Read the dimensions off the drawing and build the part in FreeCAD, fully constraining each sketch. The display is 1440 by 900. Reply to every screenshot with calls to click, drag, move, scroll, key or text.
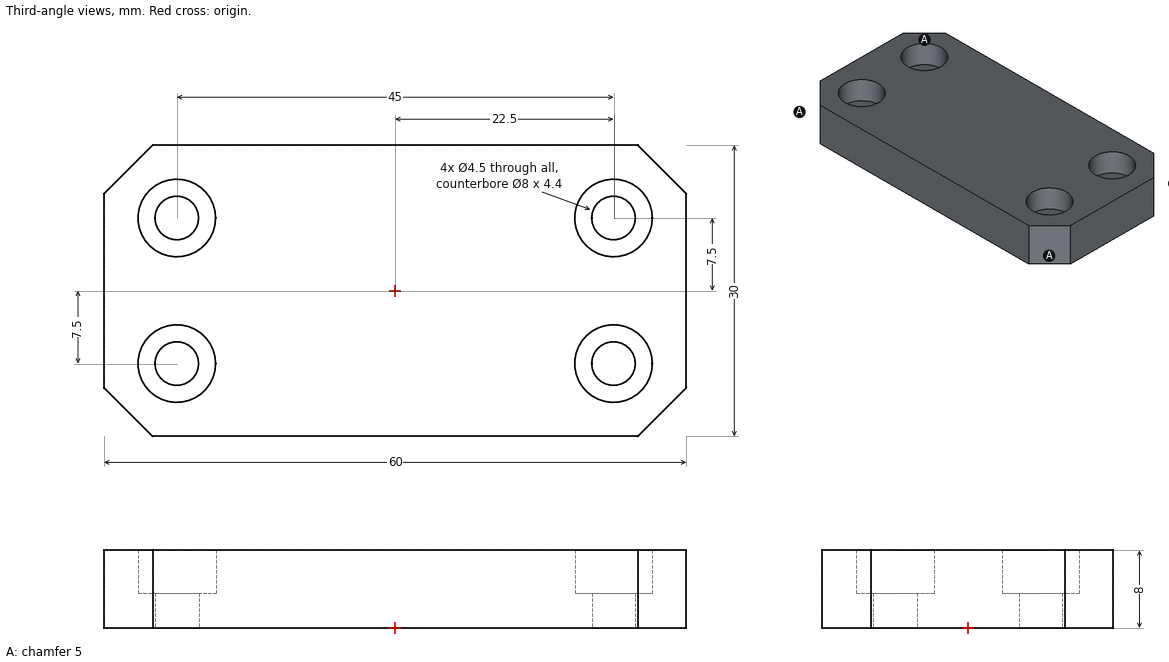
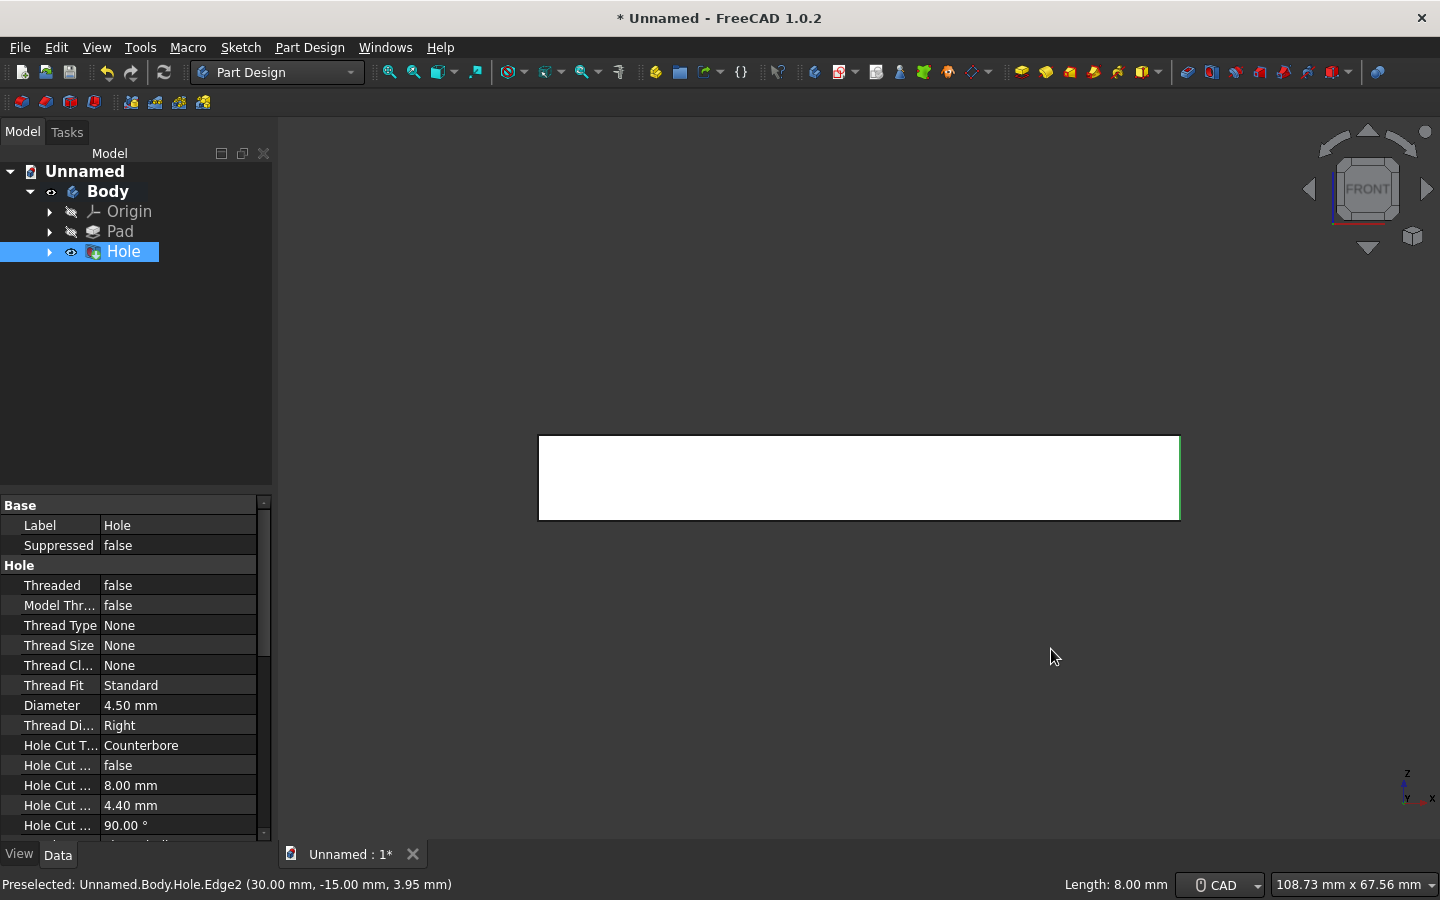
click(538, 477, ctrl)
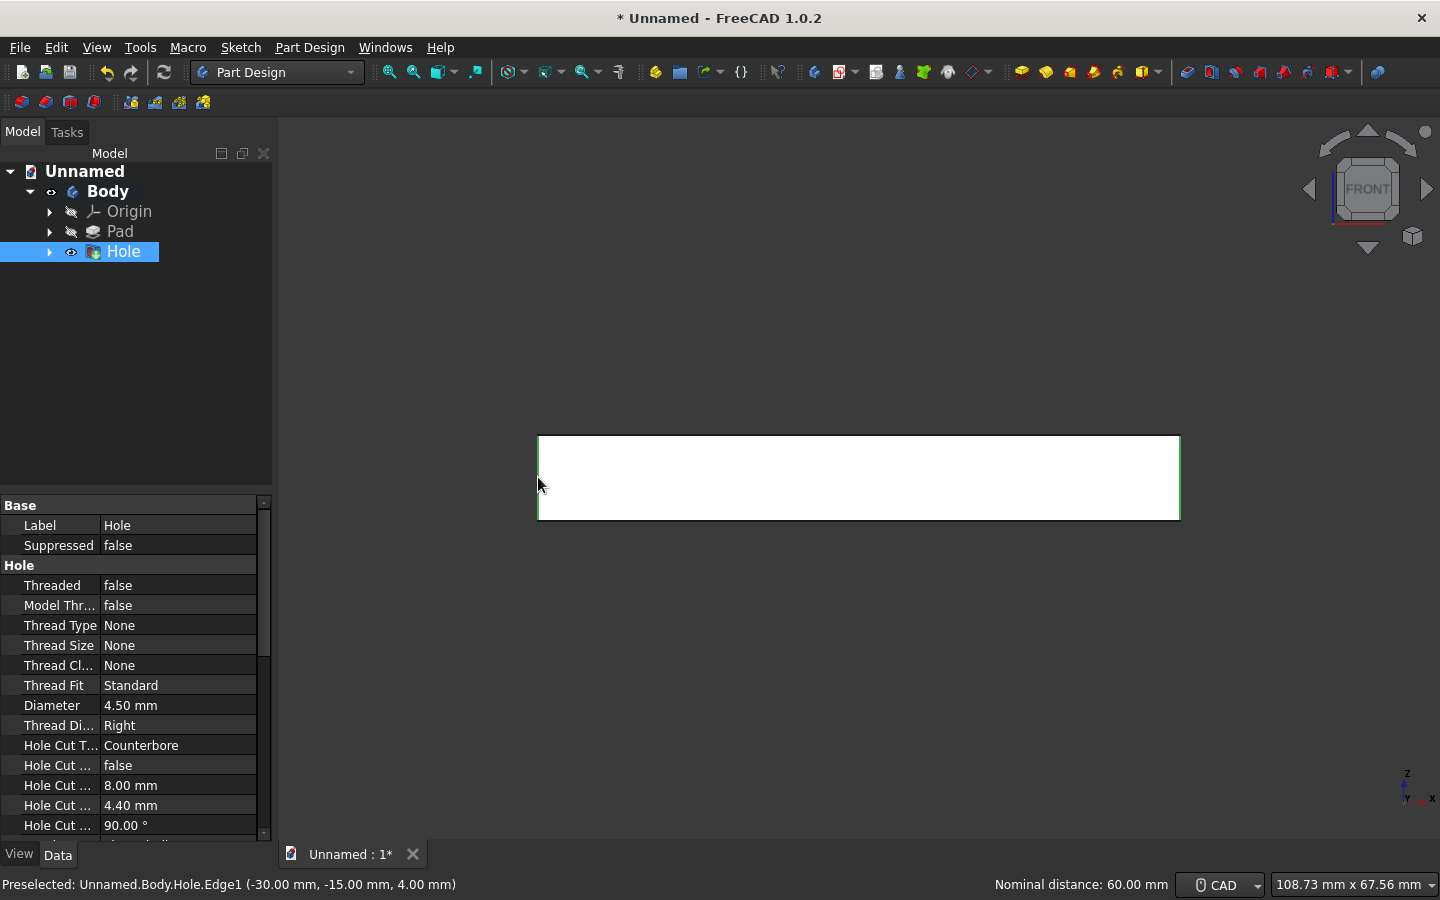
key(3)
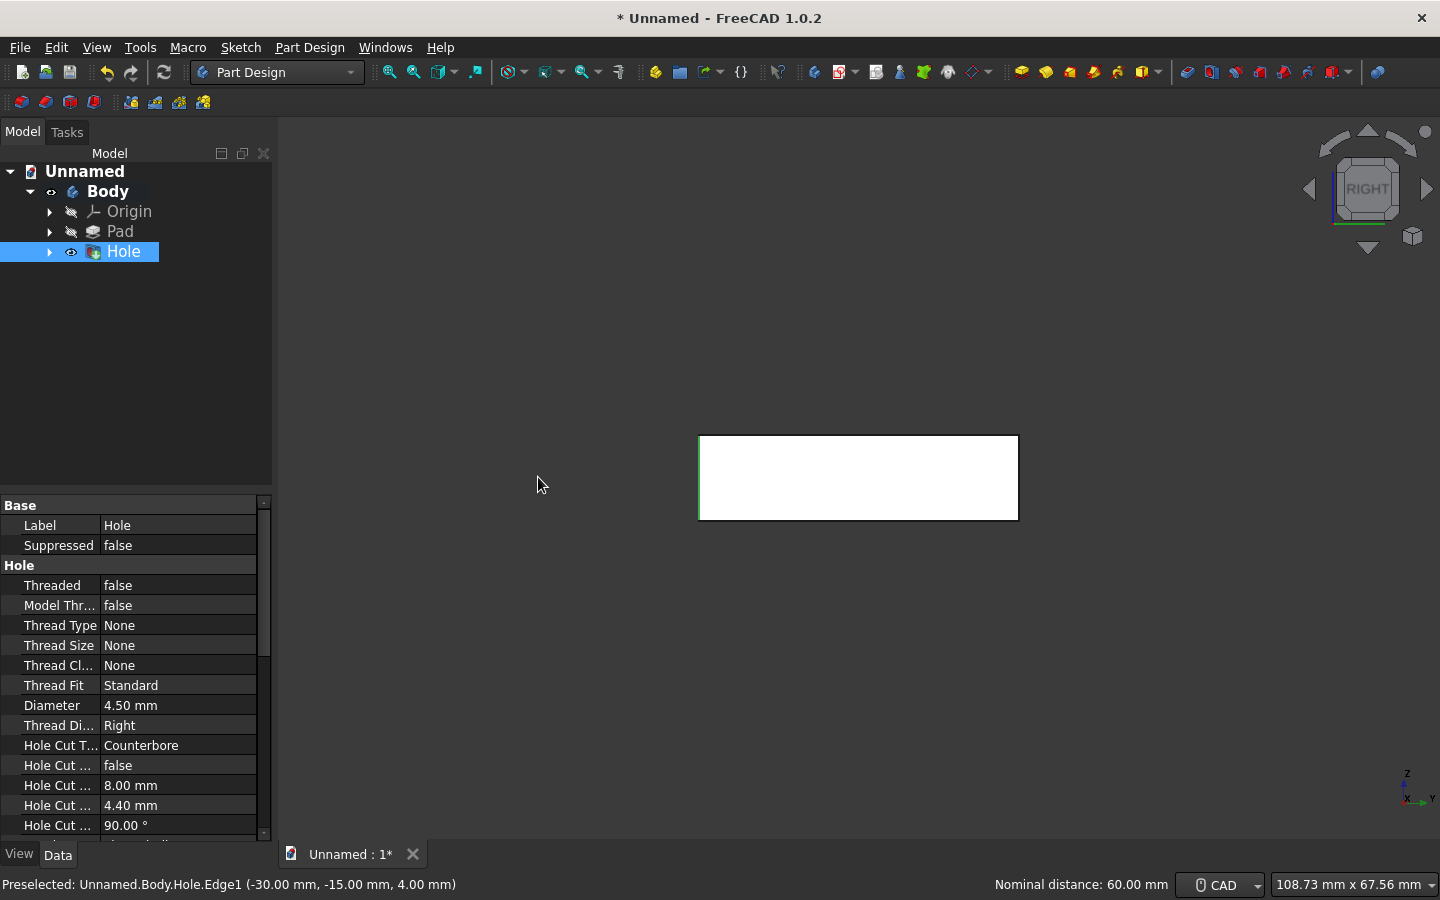
click(390, 72)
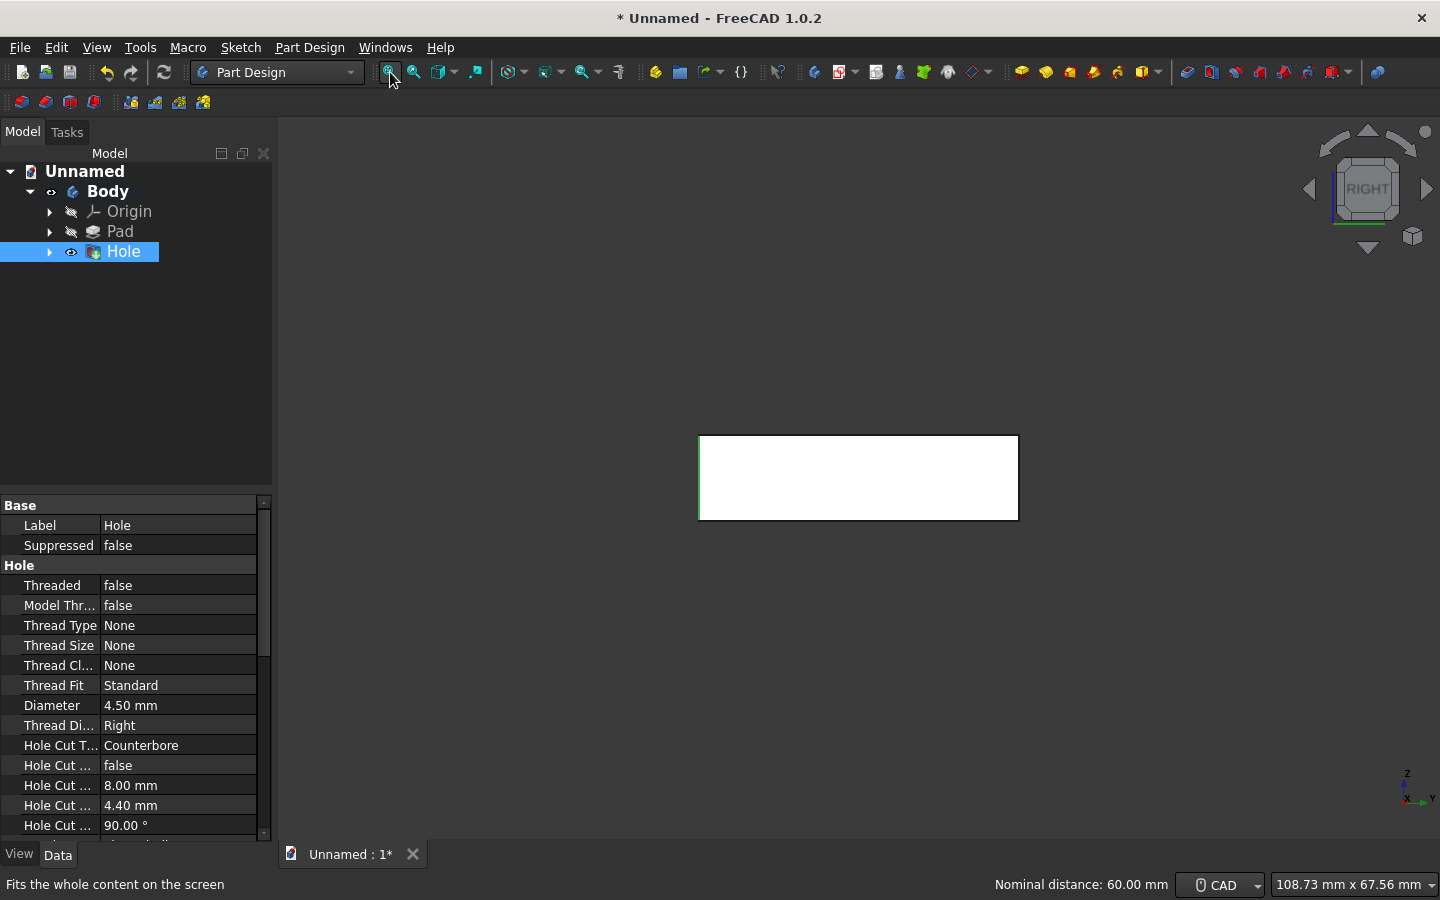
click(1019, 477, ctrl)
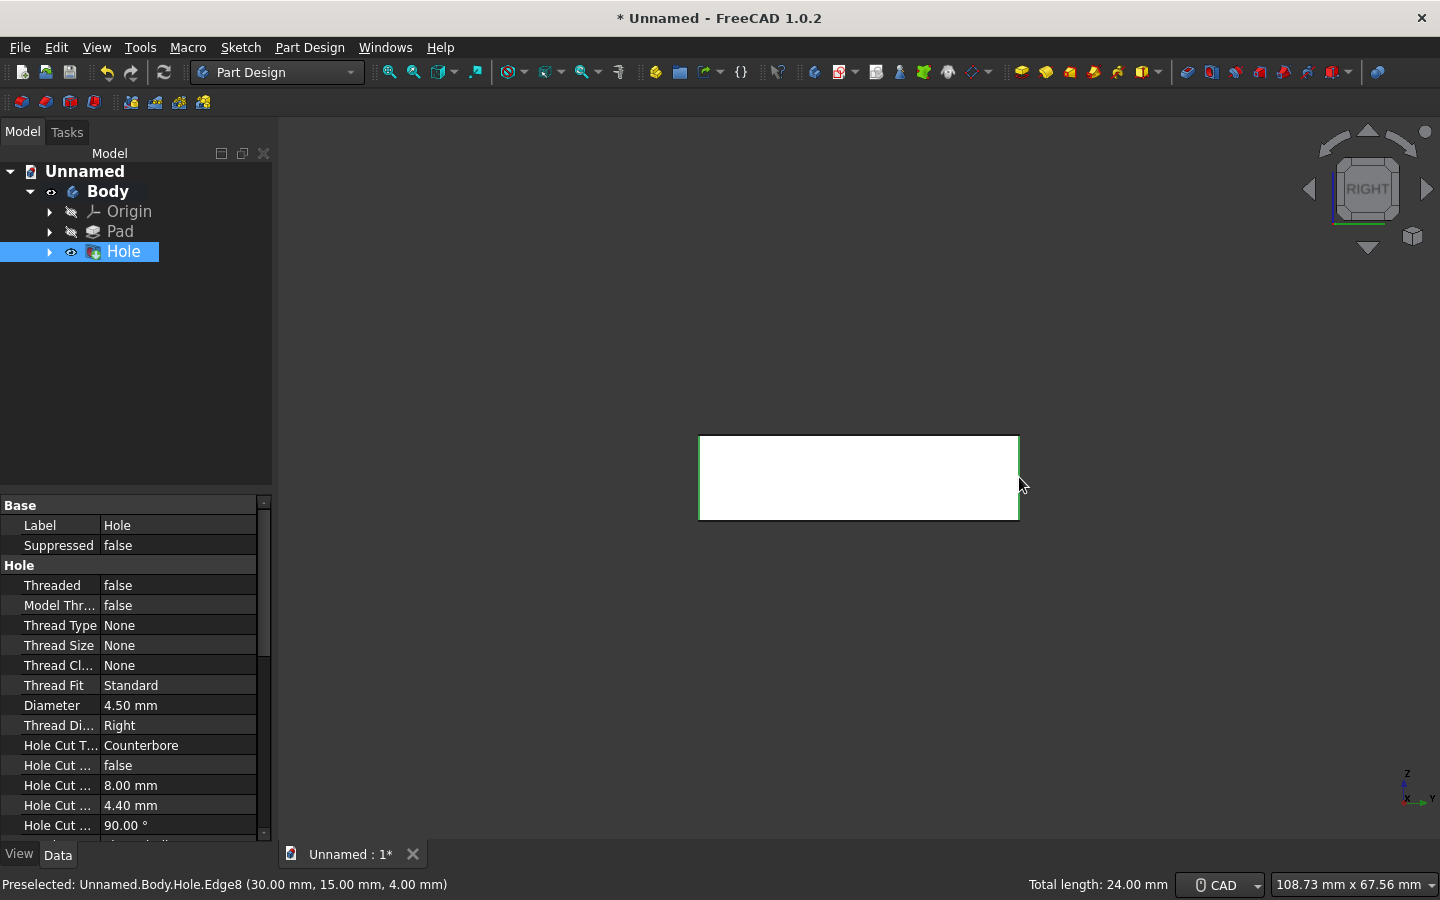
key(5)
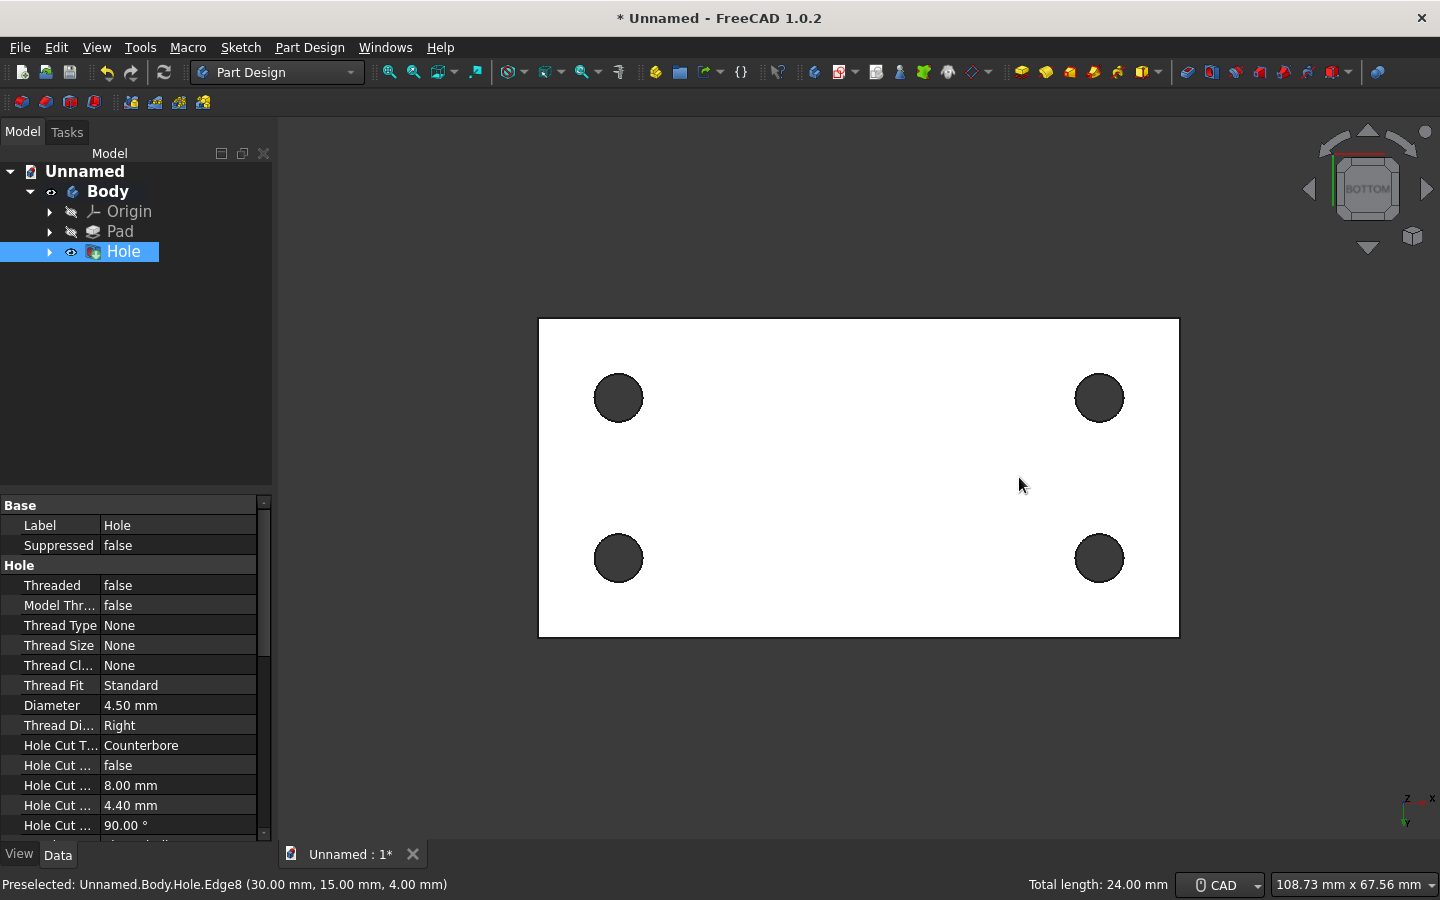
key(4)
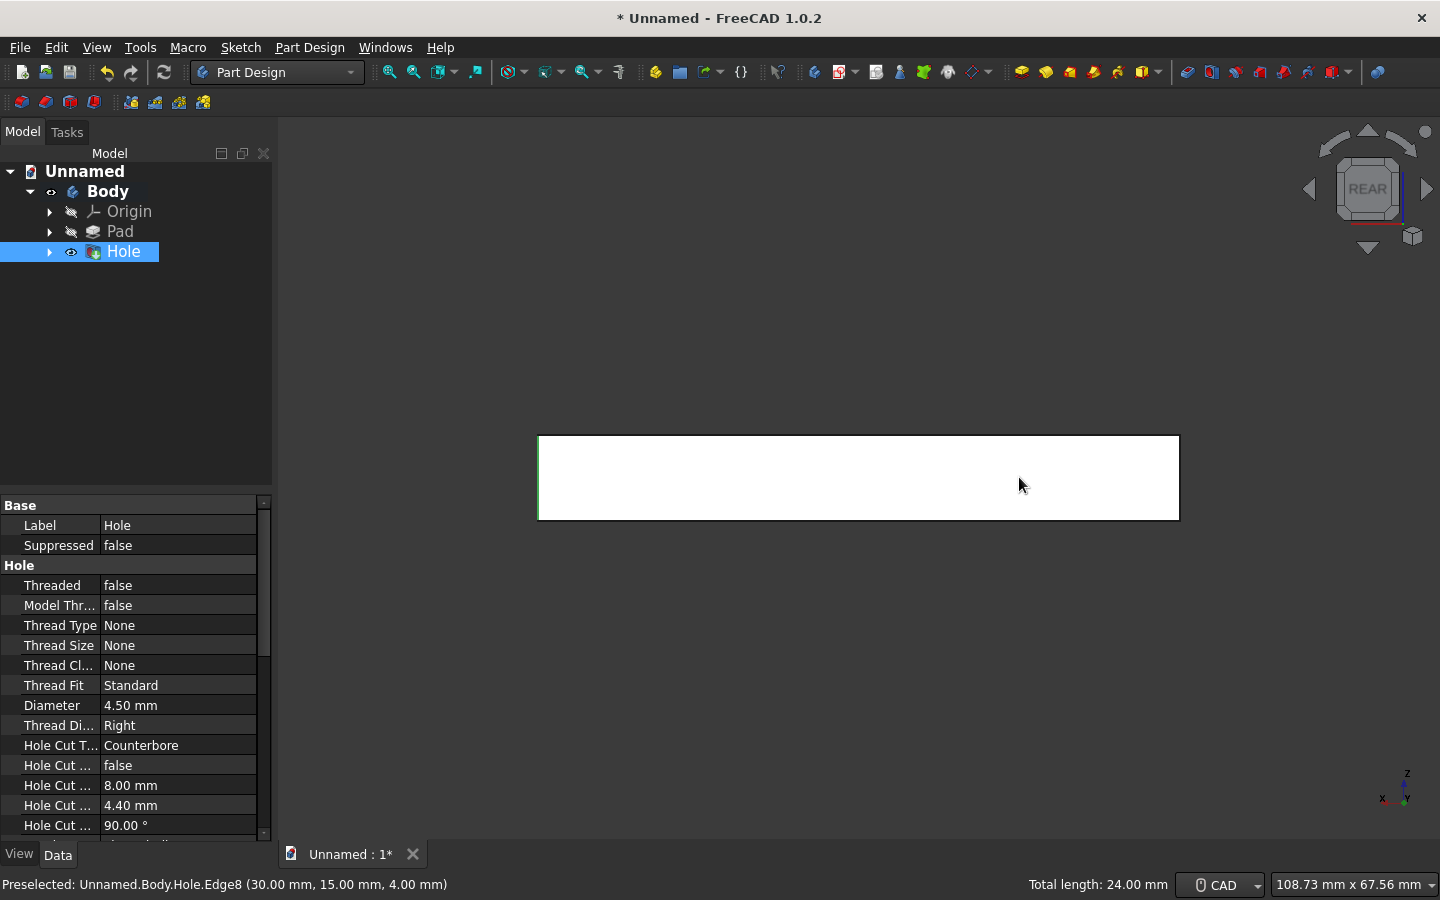
click(1180, 477, ctrl)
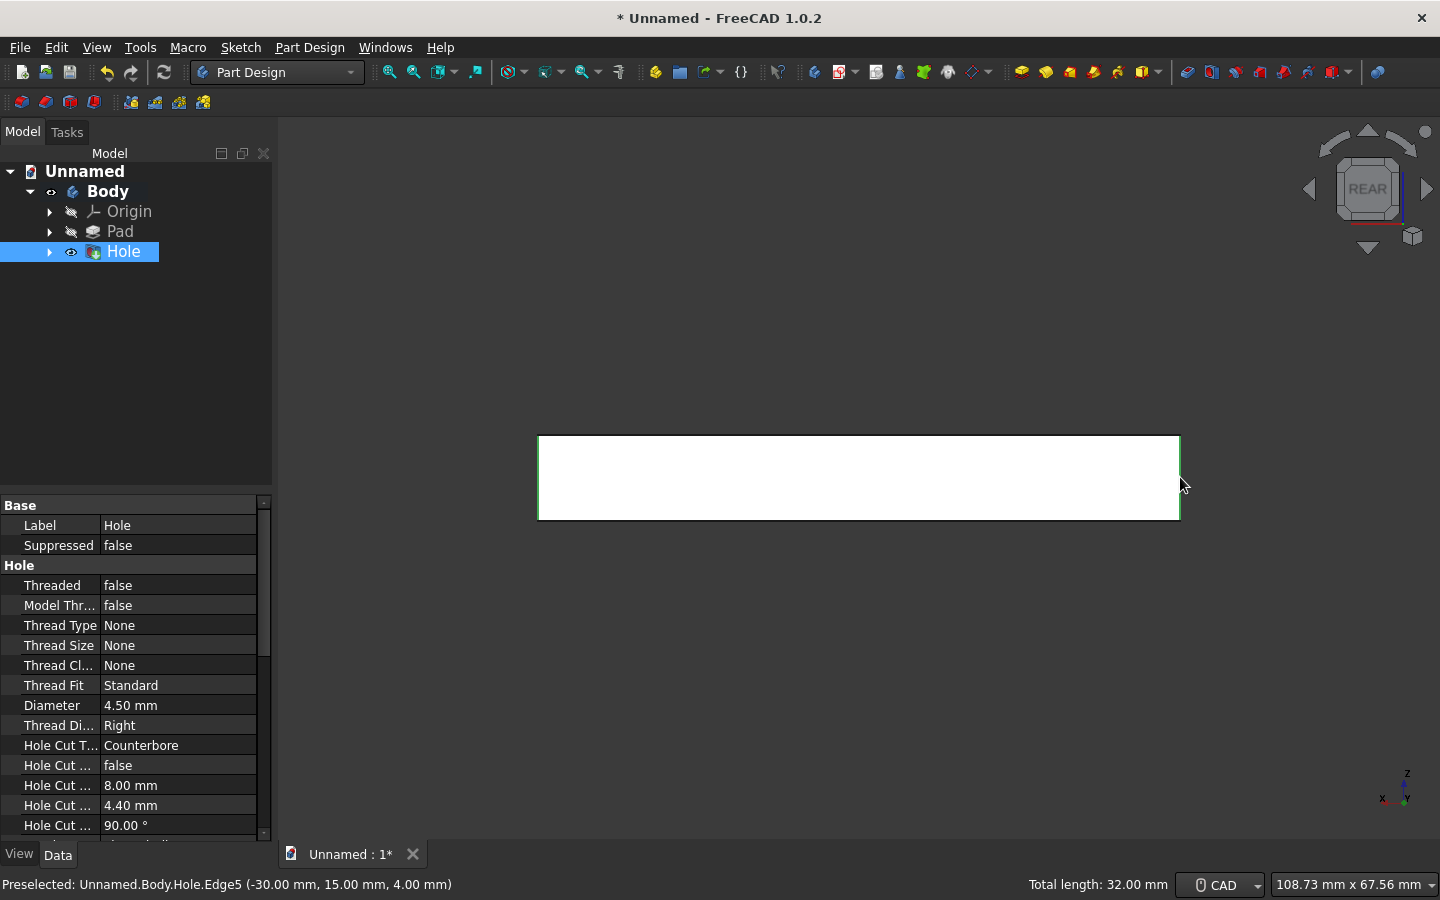
click(46, 102)